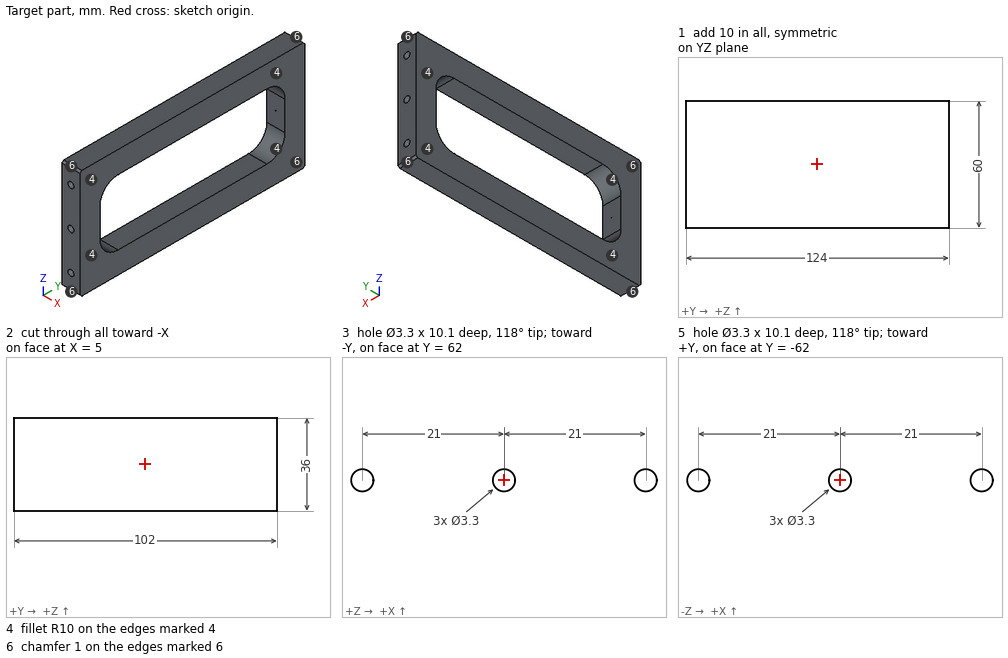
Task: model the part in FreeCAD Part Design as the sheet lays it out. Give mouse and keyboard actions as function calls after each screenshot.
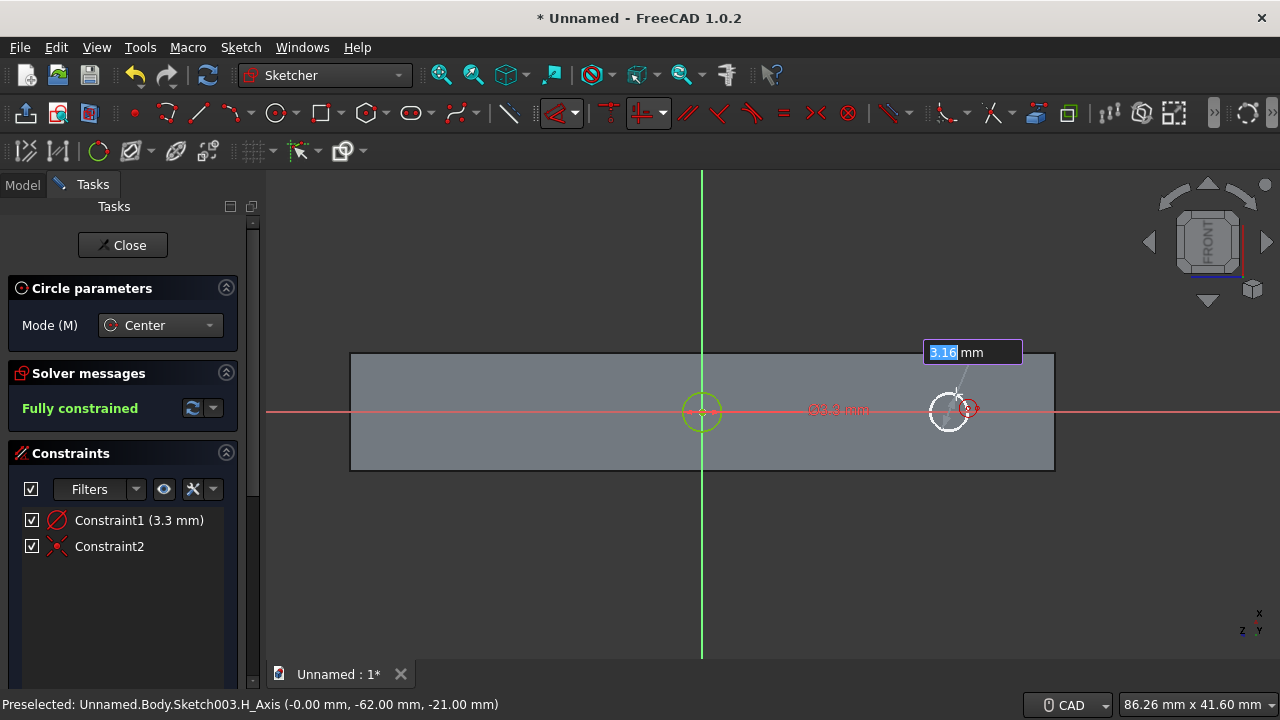
text(3.3)
key(Return)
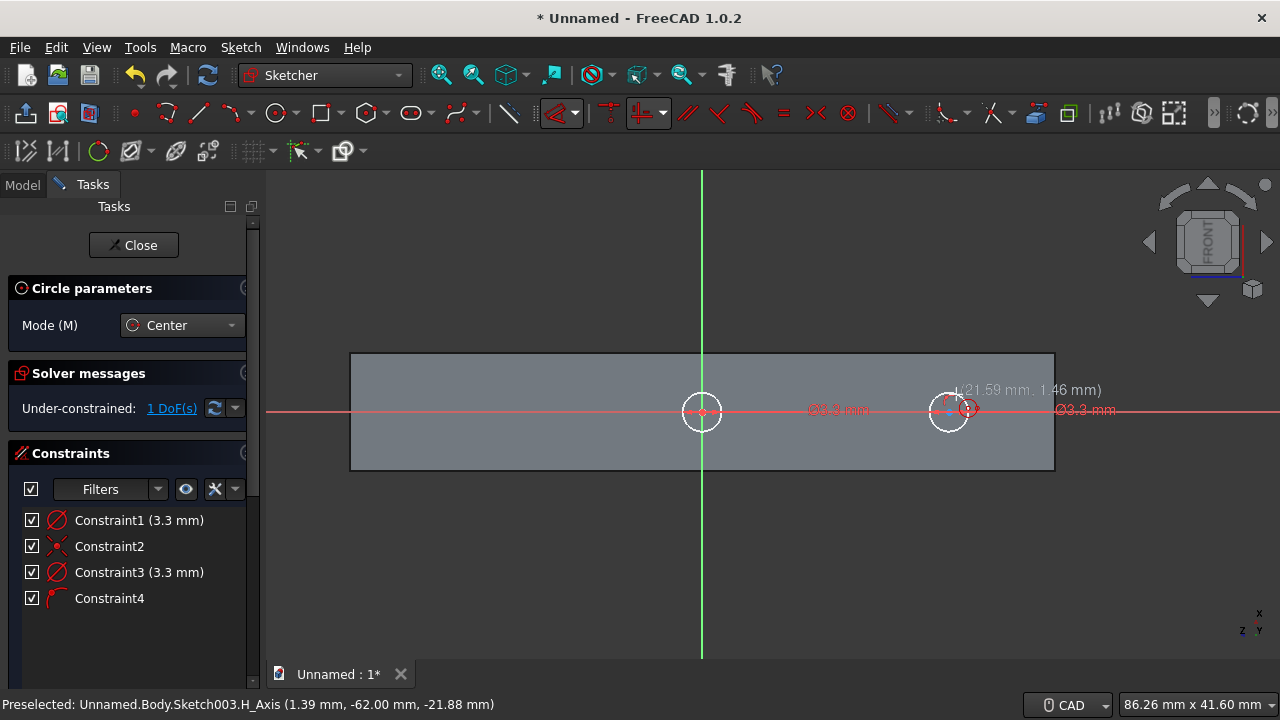
click(455, 412)
move(462, 394)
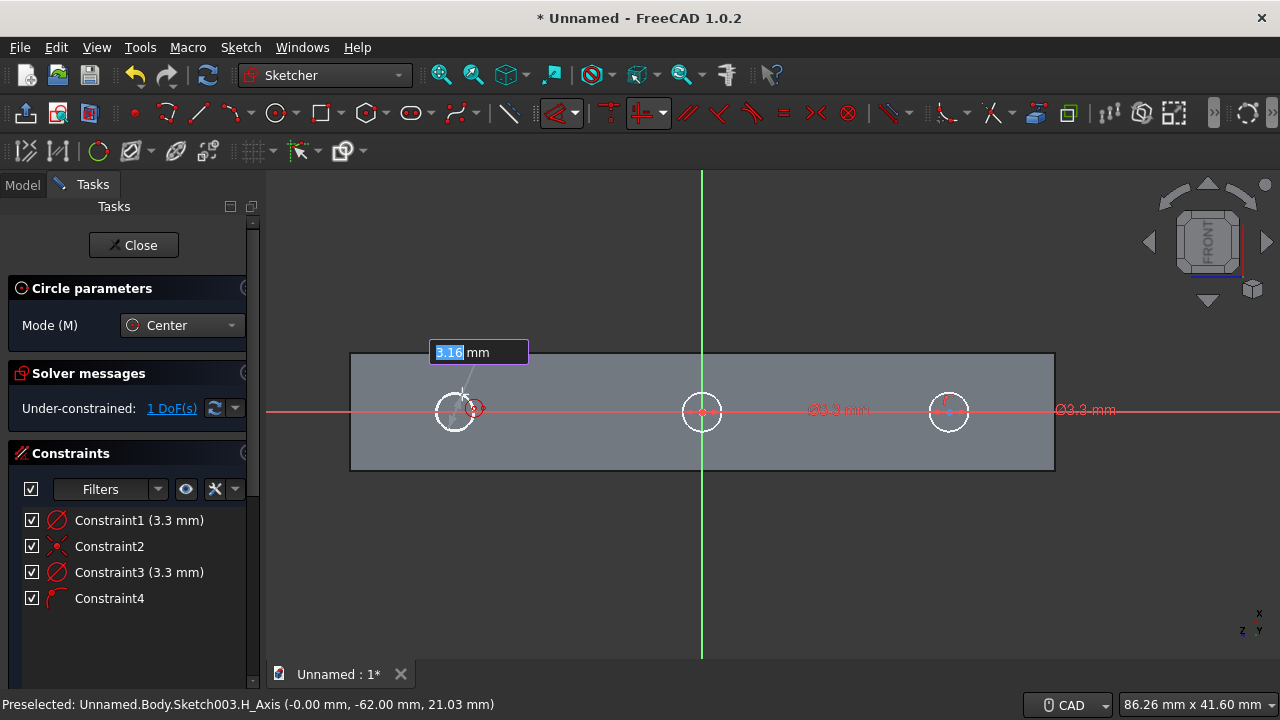
text(3.3)
key(Return)
key(Escape)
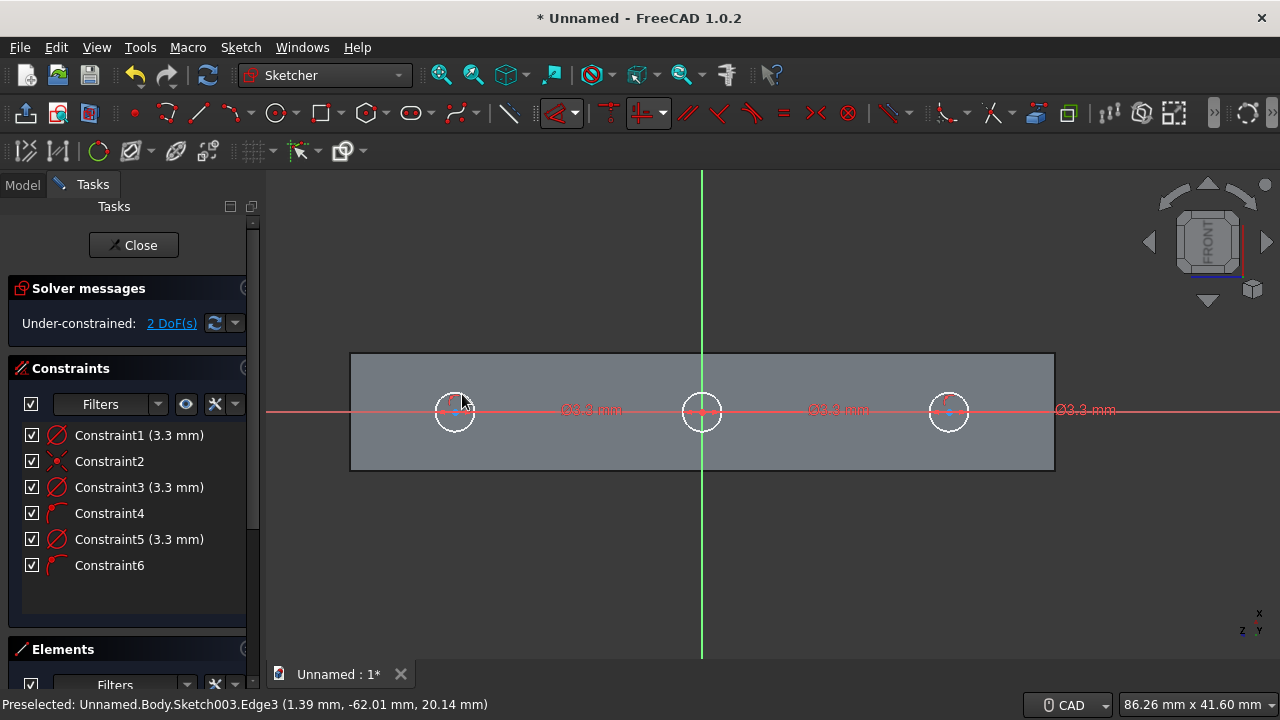
click(949, 412)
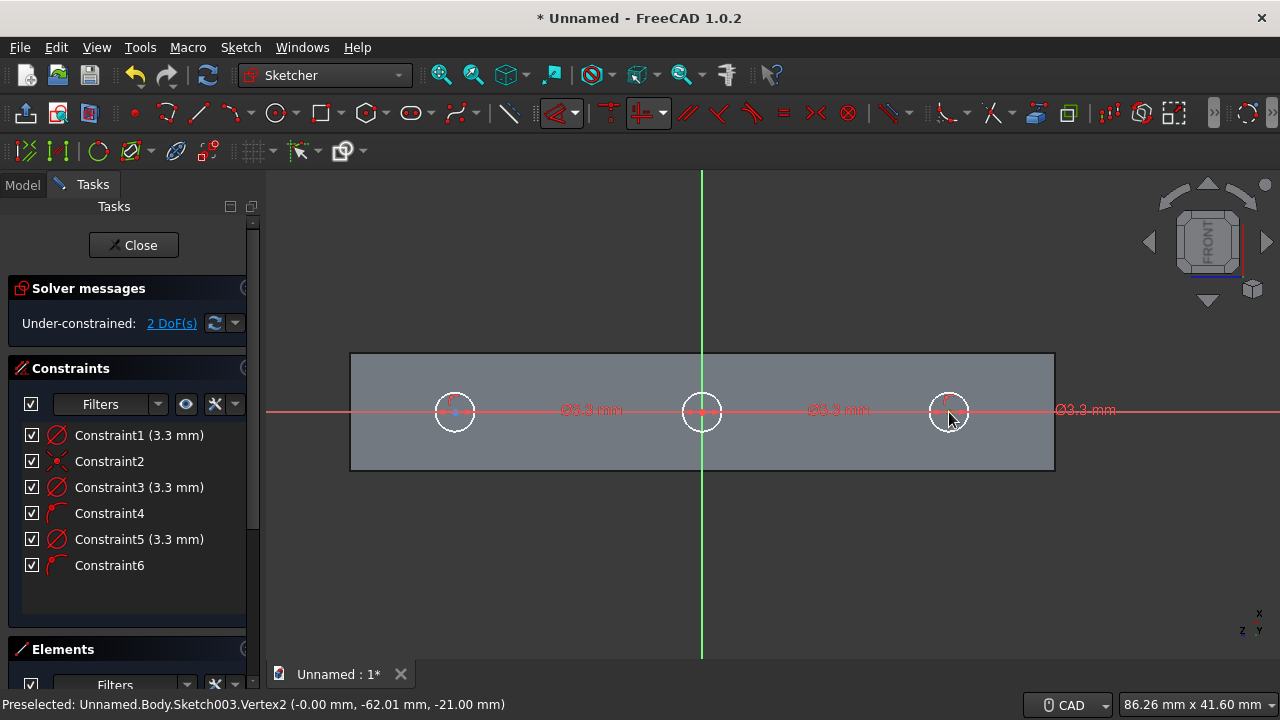
key(l)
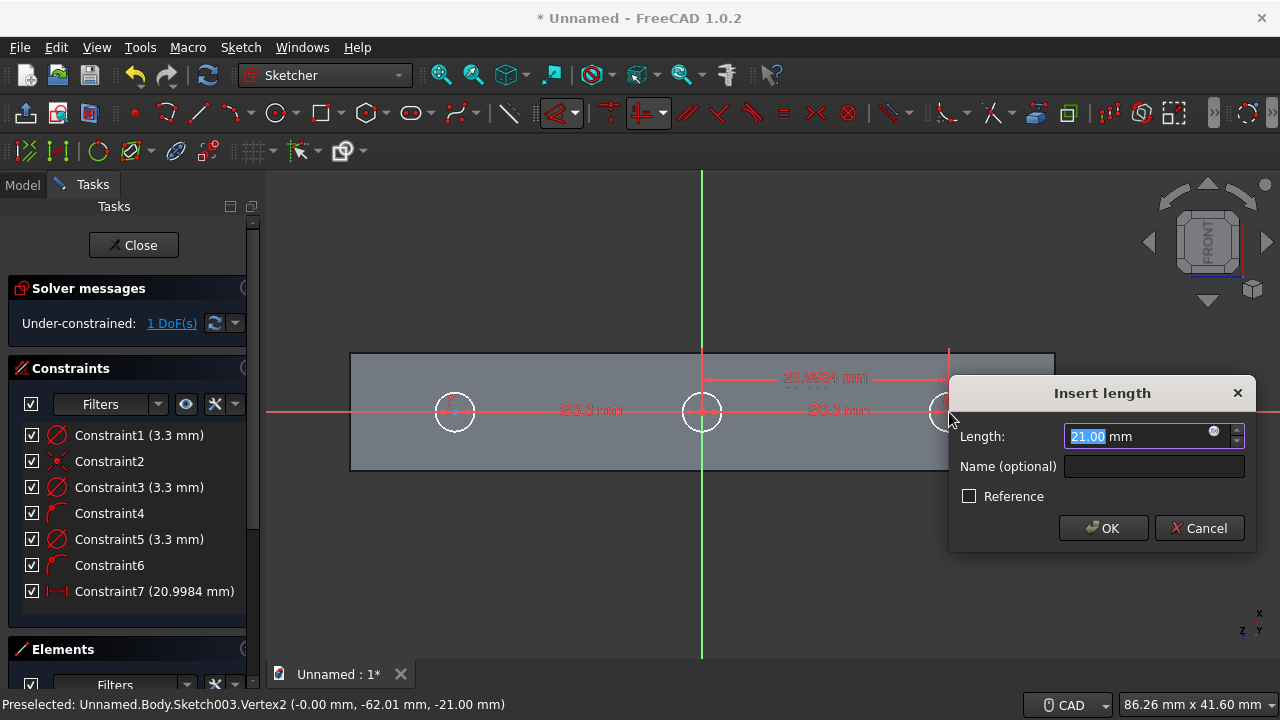
text(21)
key(Return)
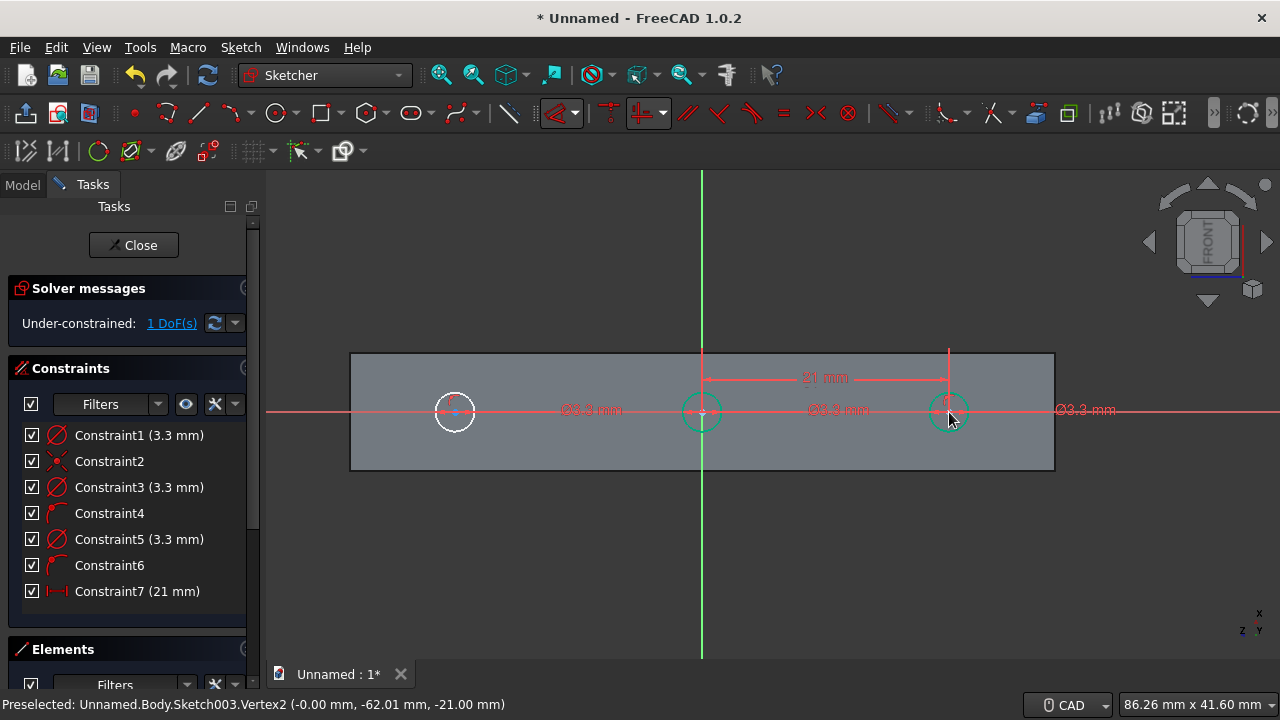
click(455, 412)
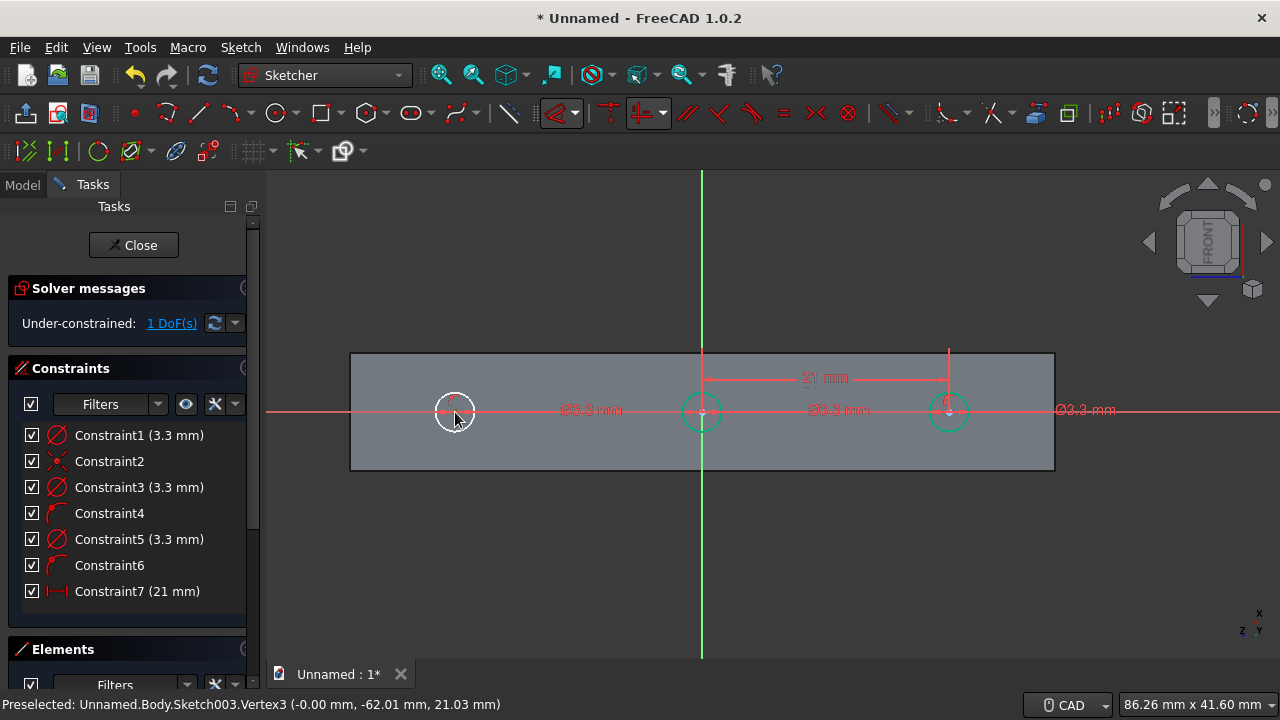
key(l)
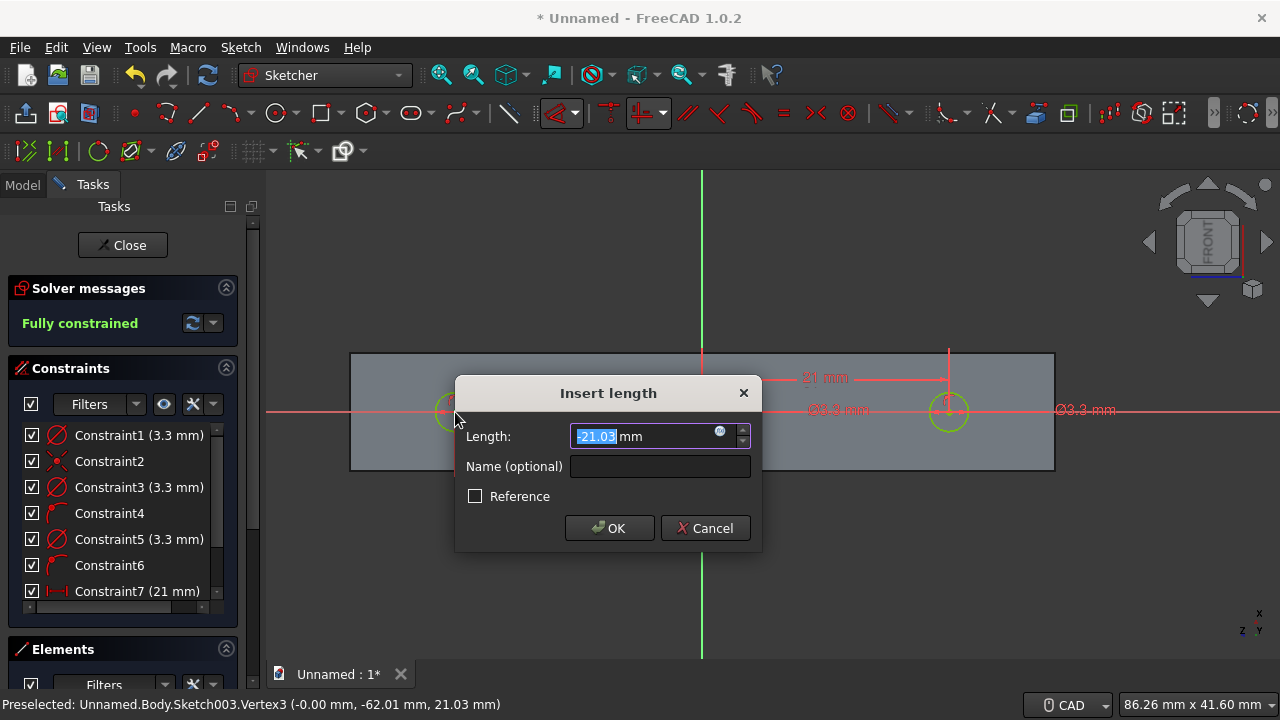
text(-21)
key(Return)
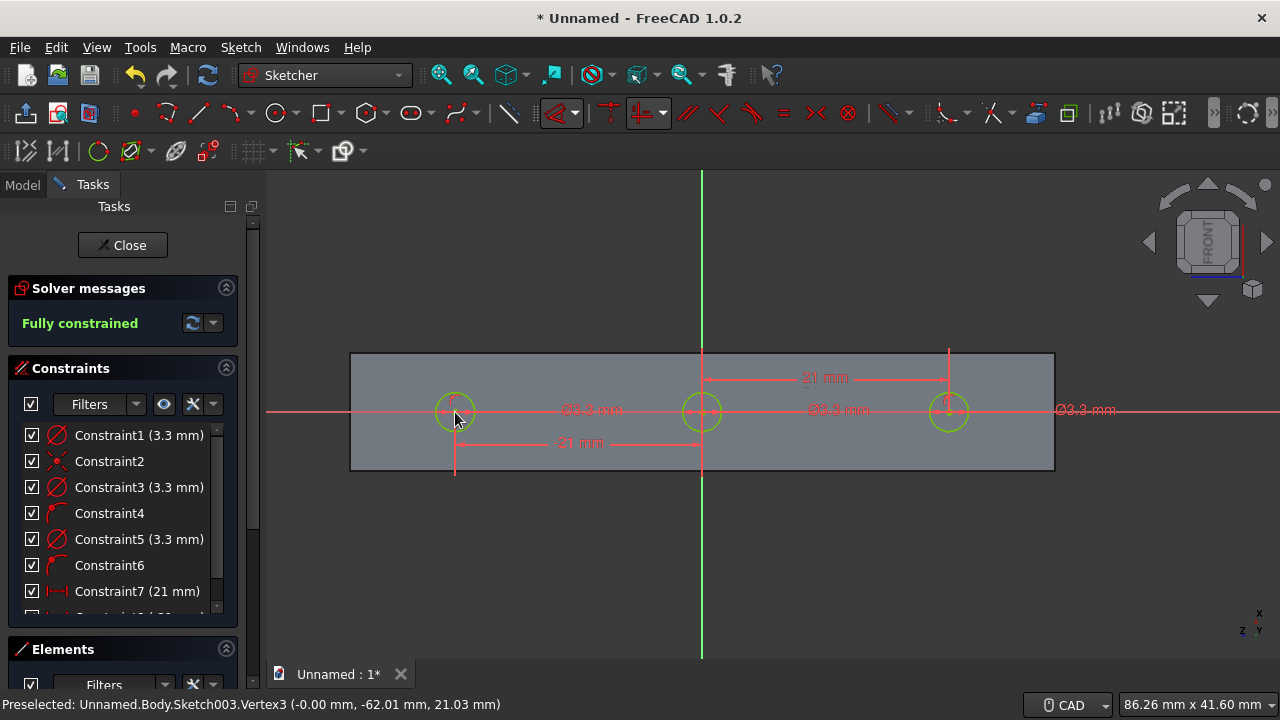
click(123, 245)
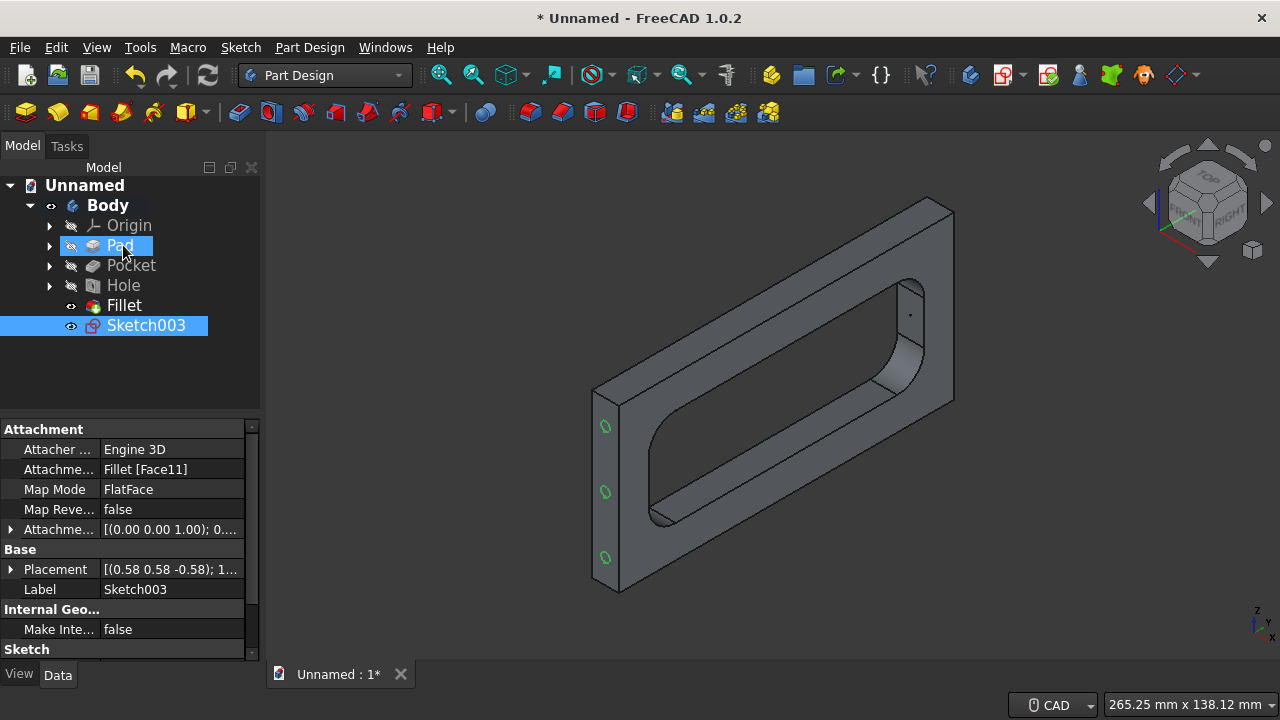
click(272, 112)